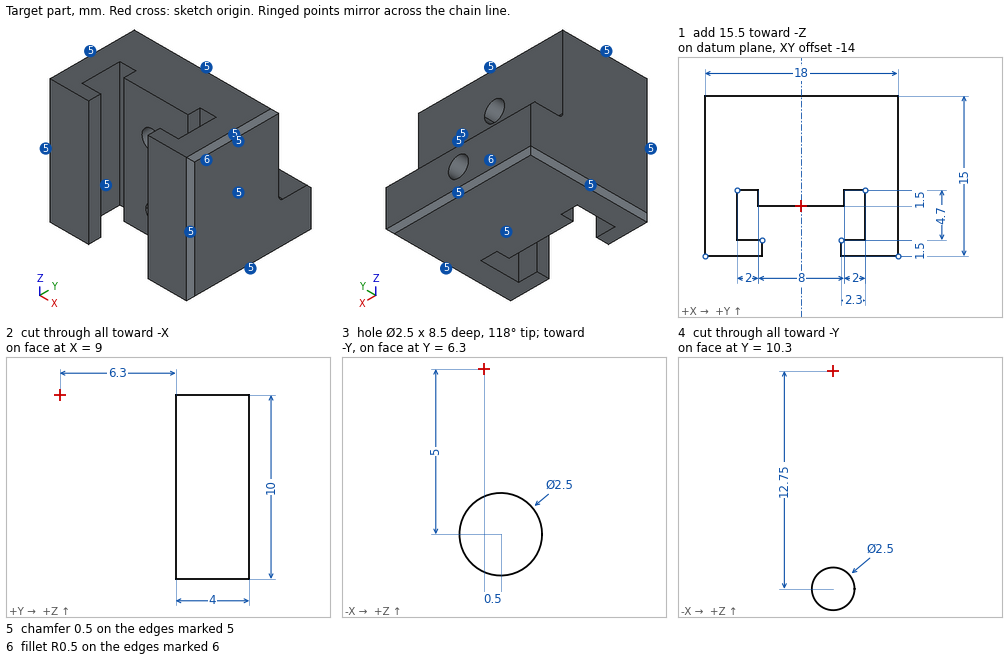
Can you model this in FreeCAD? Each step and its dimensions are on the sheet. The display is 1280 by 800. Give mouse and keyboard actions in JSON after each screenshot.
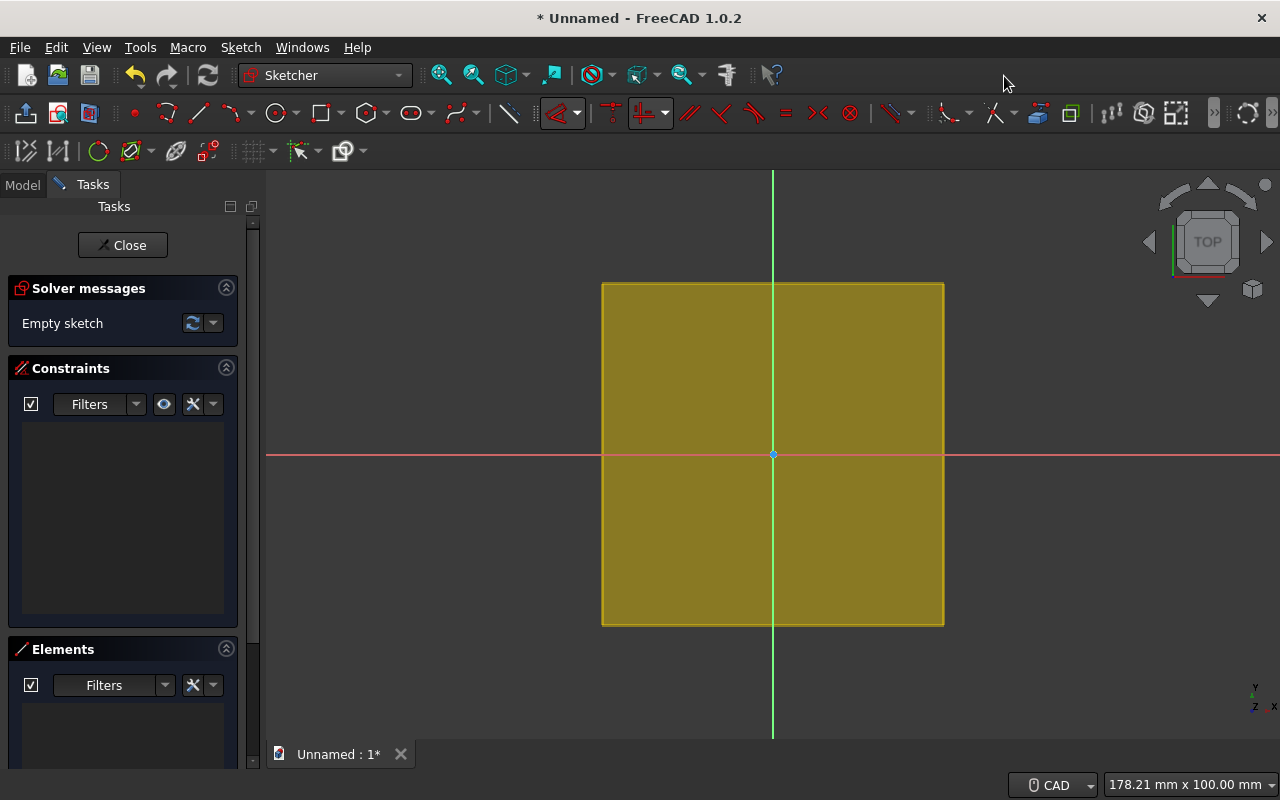
{"action": "scroll", "coordinate": [795, 433], "scroll_direction": "up", "scroll_amount": 7}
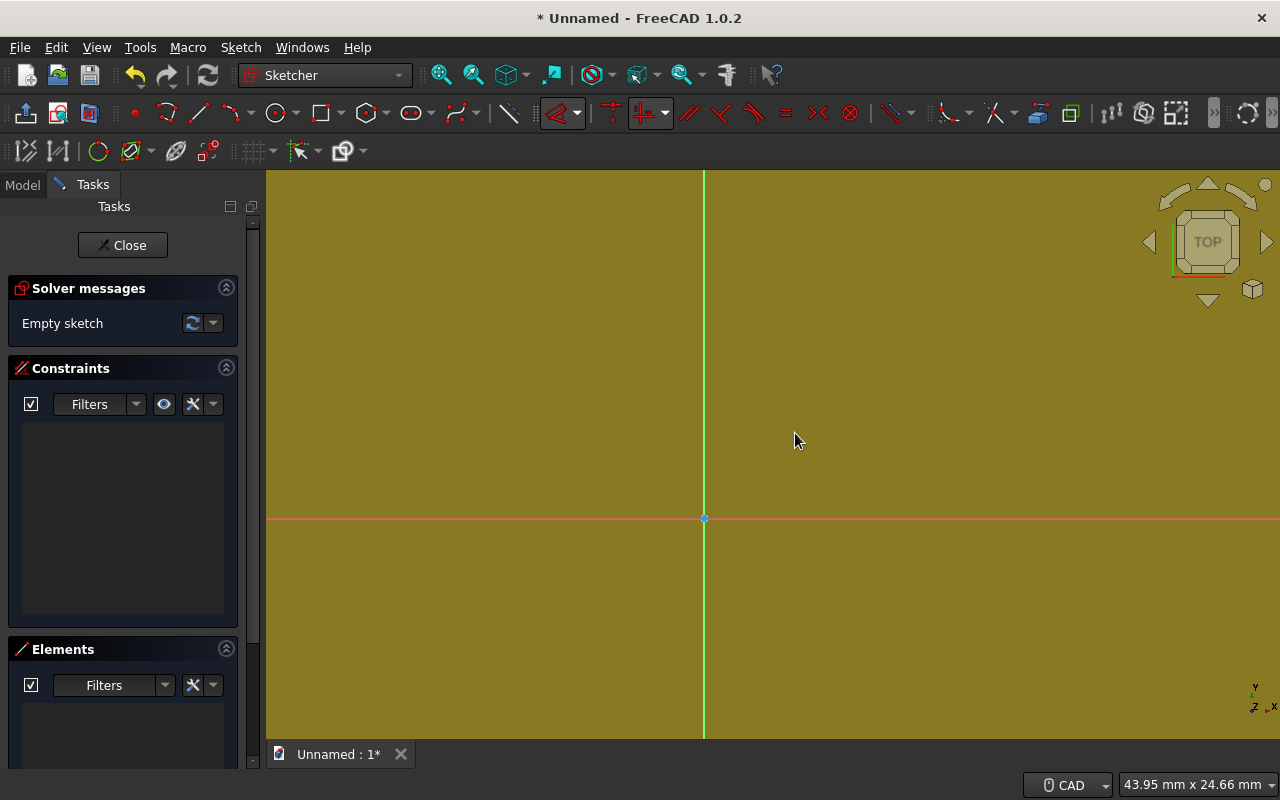
{"action": "left_click", "coordinate": [168, 114]}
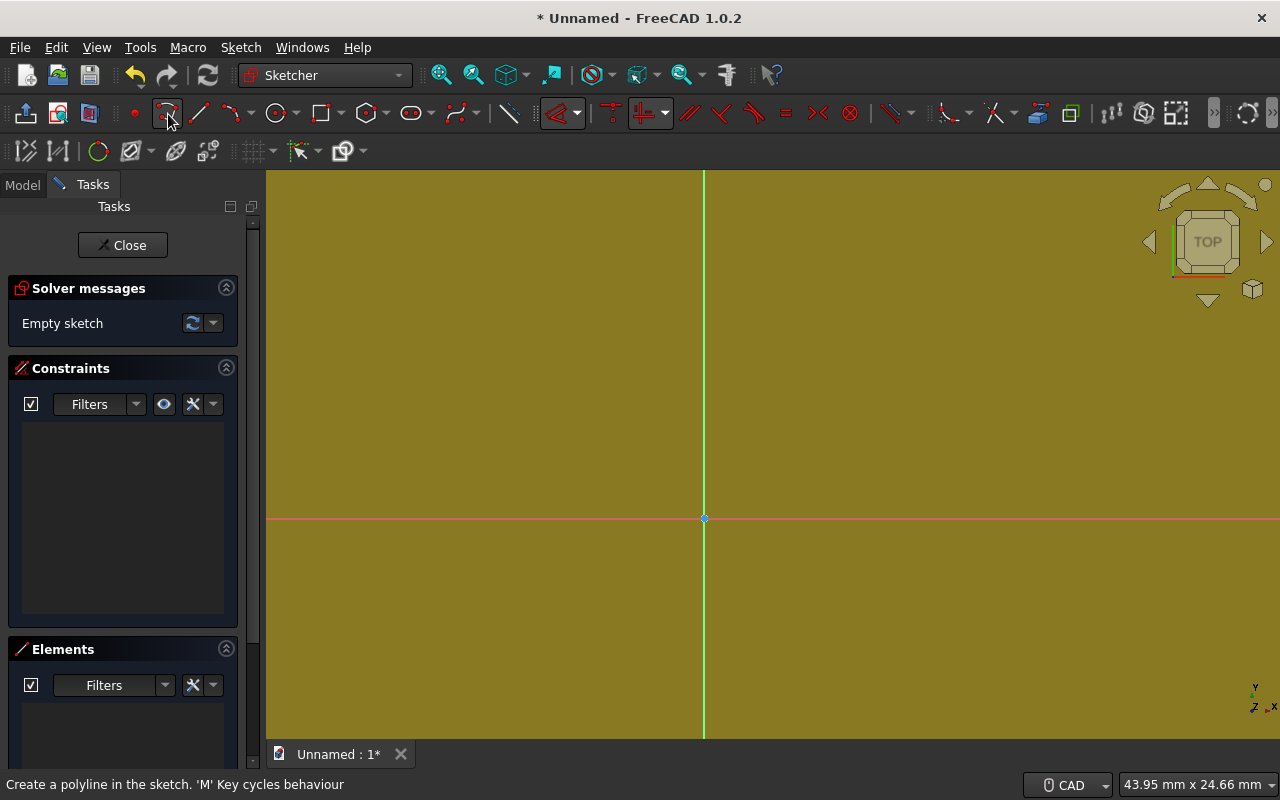
{"action": "left_click", "coordinate": [612, 519]}
{"action": "left_click", "coordinate": [796, 510]}
{"action": "left_click", "coordinate": [796, 484]}
{"action": "left_click", "coordinate": [843, 484]}
{"action": "left_click", "coordinate": [843, 593]}
{"action": "left_click", "coordinate": [790, 593]}
{"action": "left_click", "coordinate": [790, 627]}
{"action": "left_click", "coordinate": [912, 627]}
{"action": "left_click", "coordinate": [912, 281]}
{"action": "left_click", "coordinate": [497, 281]}
{"action": "left_click", "coordinate": [497, 627]}
{"action": "left_click", "coordinate": [619, 627]}
{"action": "left_click", "coordinate": [619, 593]}
{"action": "left_click", "coordinate": [566, 593]}
{"action": "left_click", "coordinate": [566, 484]}
{"action": "left_click", "coordinate": [612, 484]}
{"action": "left_click", "coordinate": [612, 519]}
{"action": "key", "text": "Escape"}
{"action": "key", "text": "Escape"}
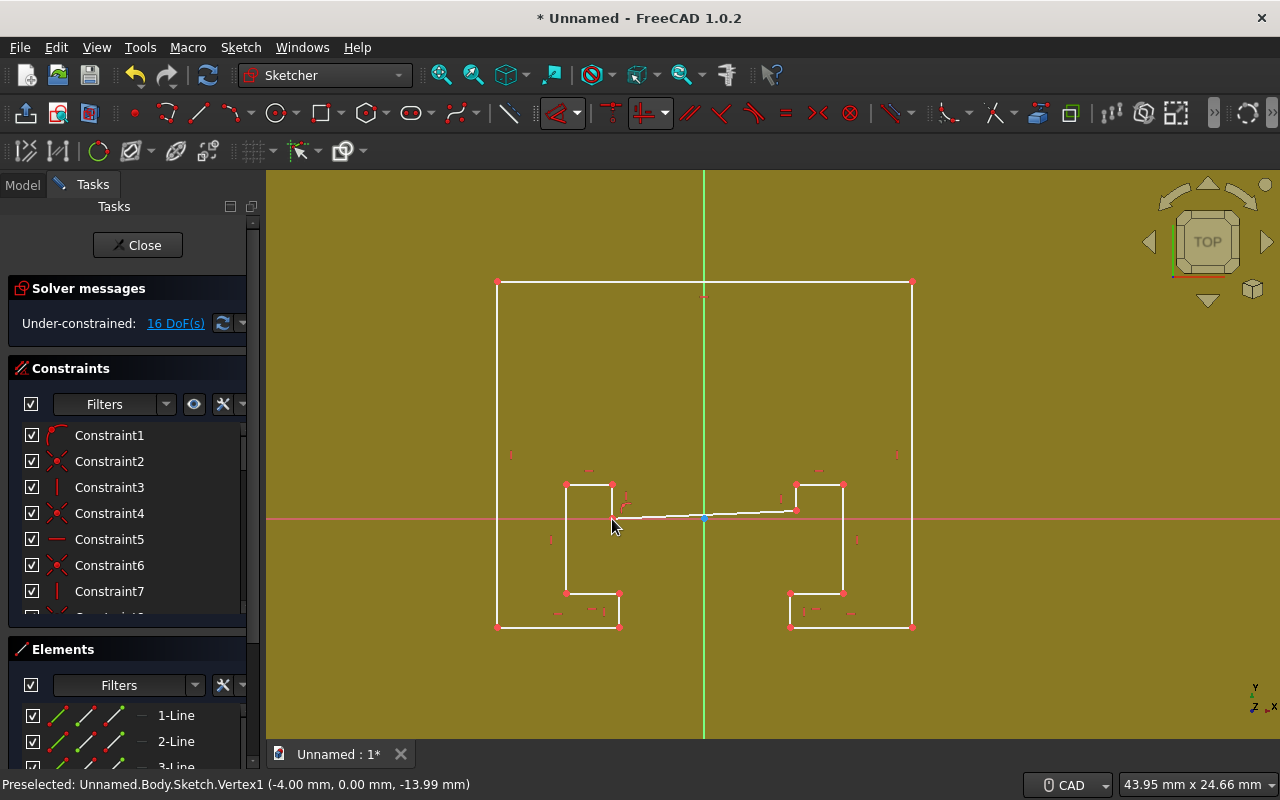
{"action": "left_click", "coordinate": [667, 516]}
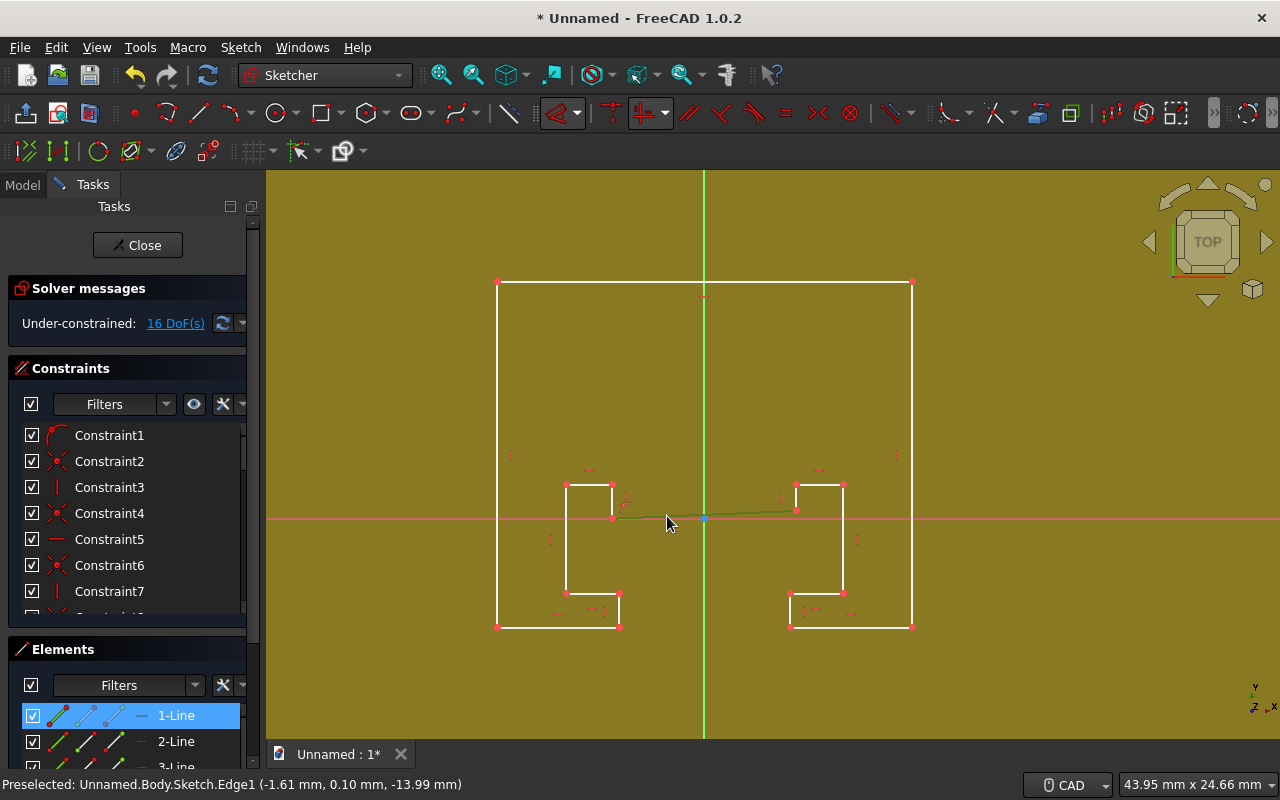
{"action": "key", "text": "h"}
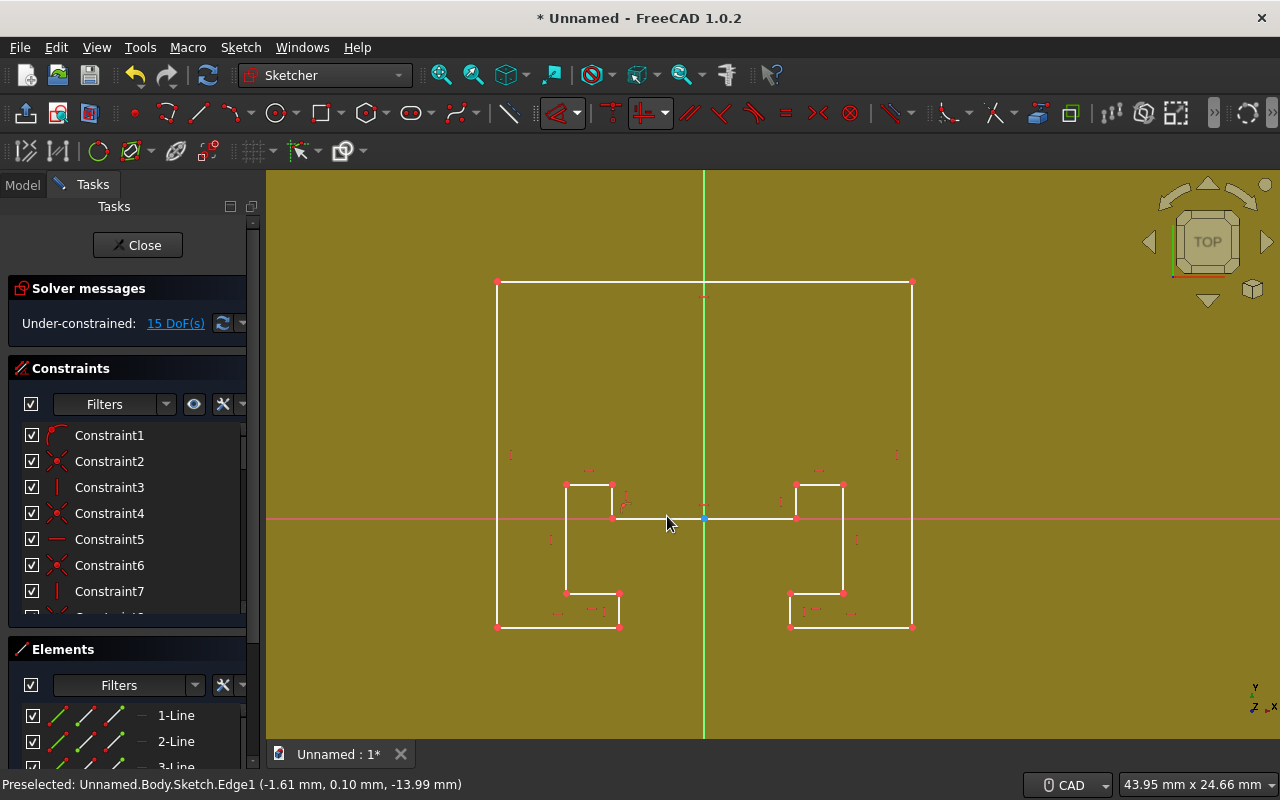
{"action": "left_click", "coordinate": [912, 628]}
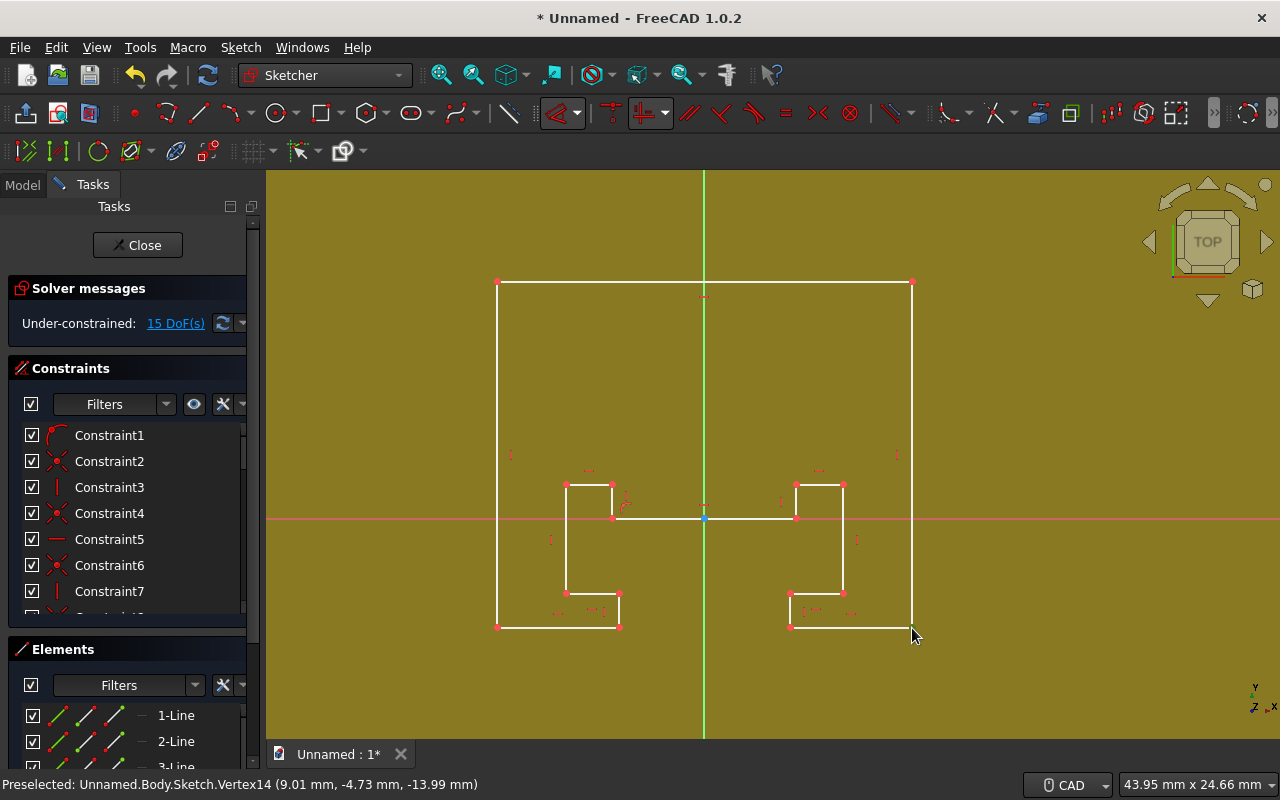
{"action": "left_click", "coordinate": [497, 628]}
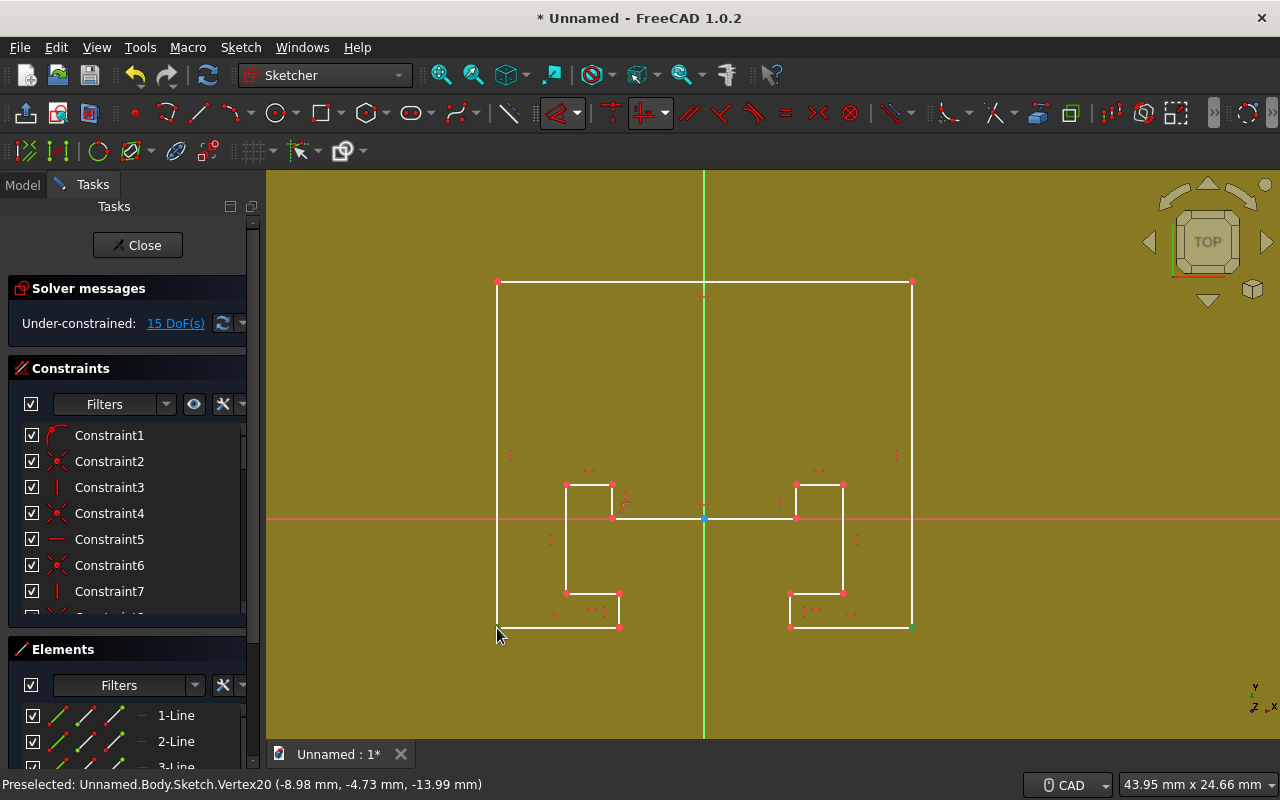
{"action": "left_click", "coordinate": [704, 674]}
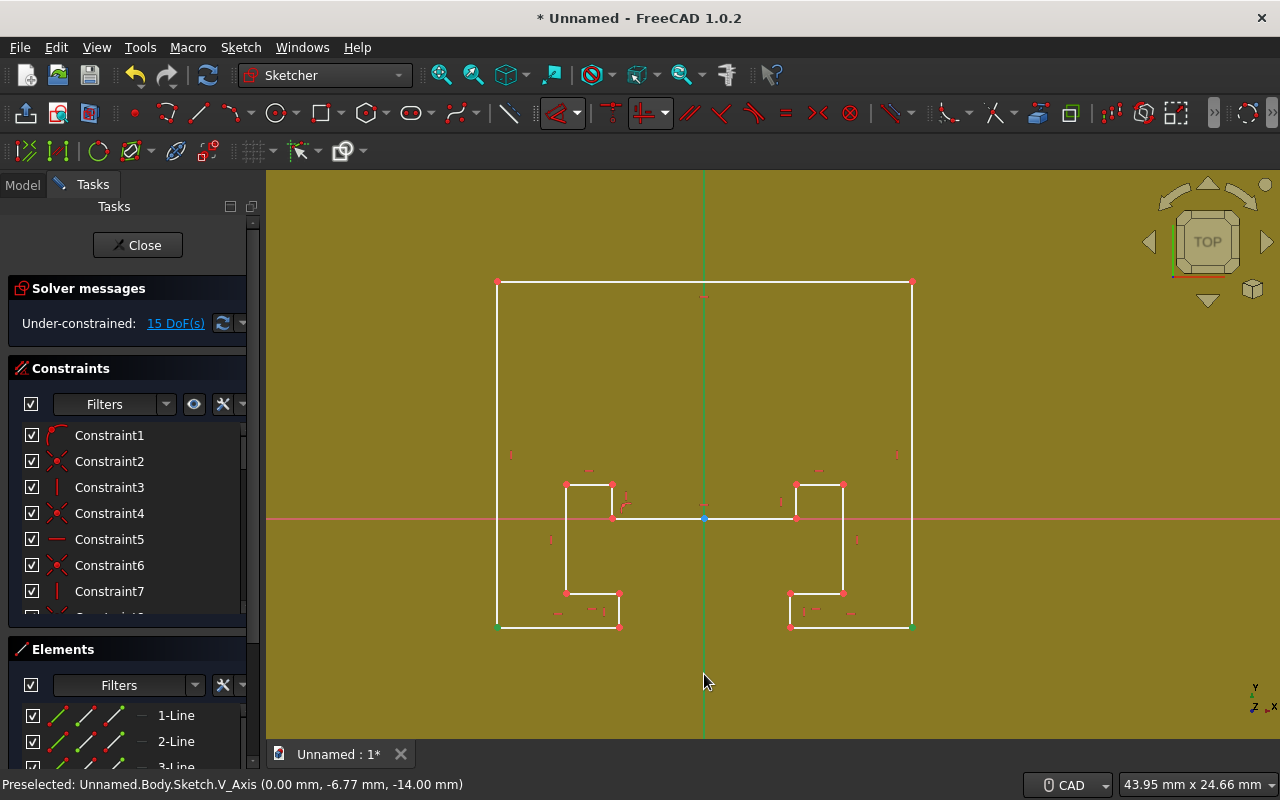
{"action": "key", "text": "s"}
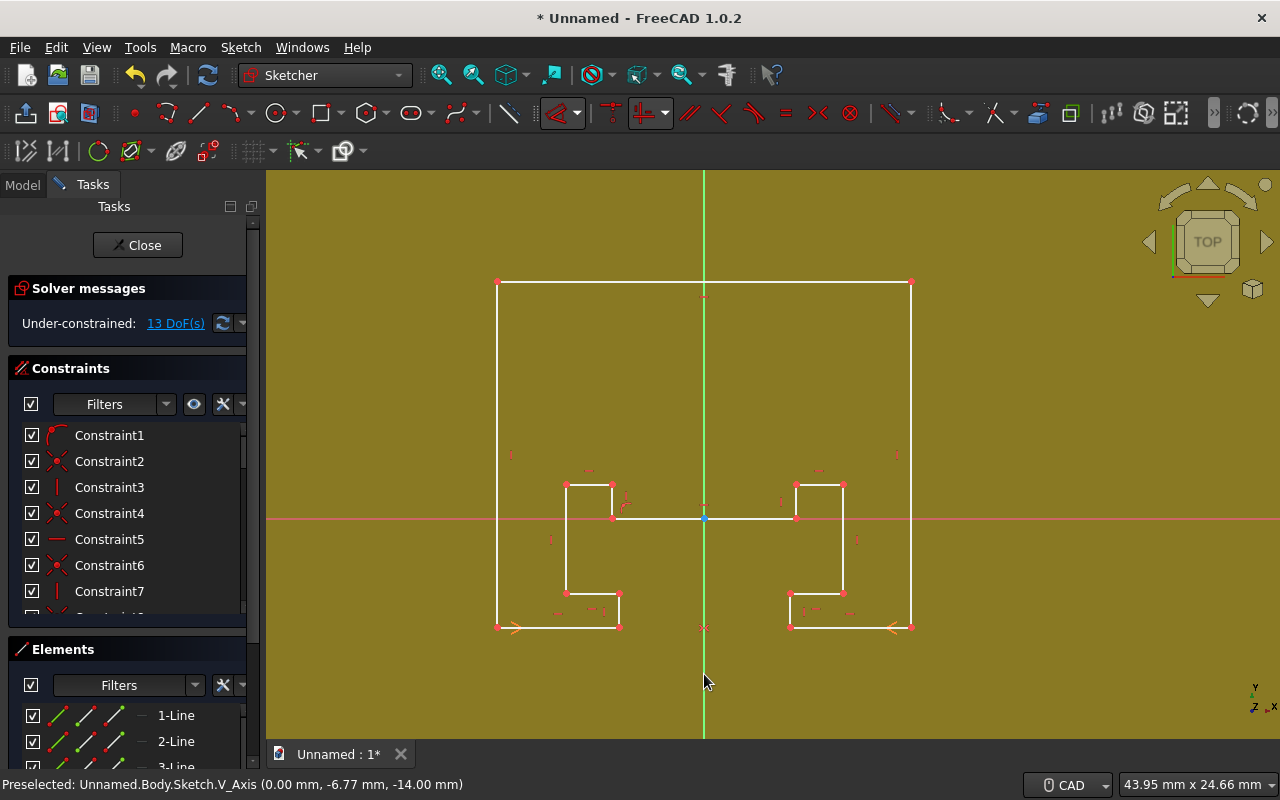
{"action": "left_click", "coordinate": [790, 594]}